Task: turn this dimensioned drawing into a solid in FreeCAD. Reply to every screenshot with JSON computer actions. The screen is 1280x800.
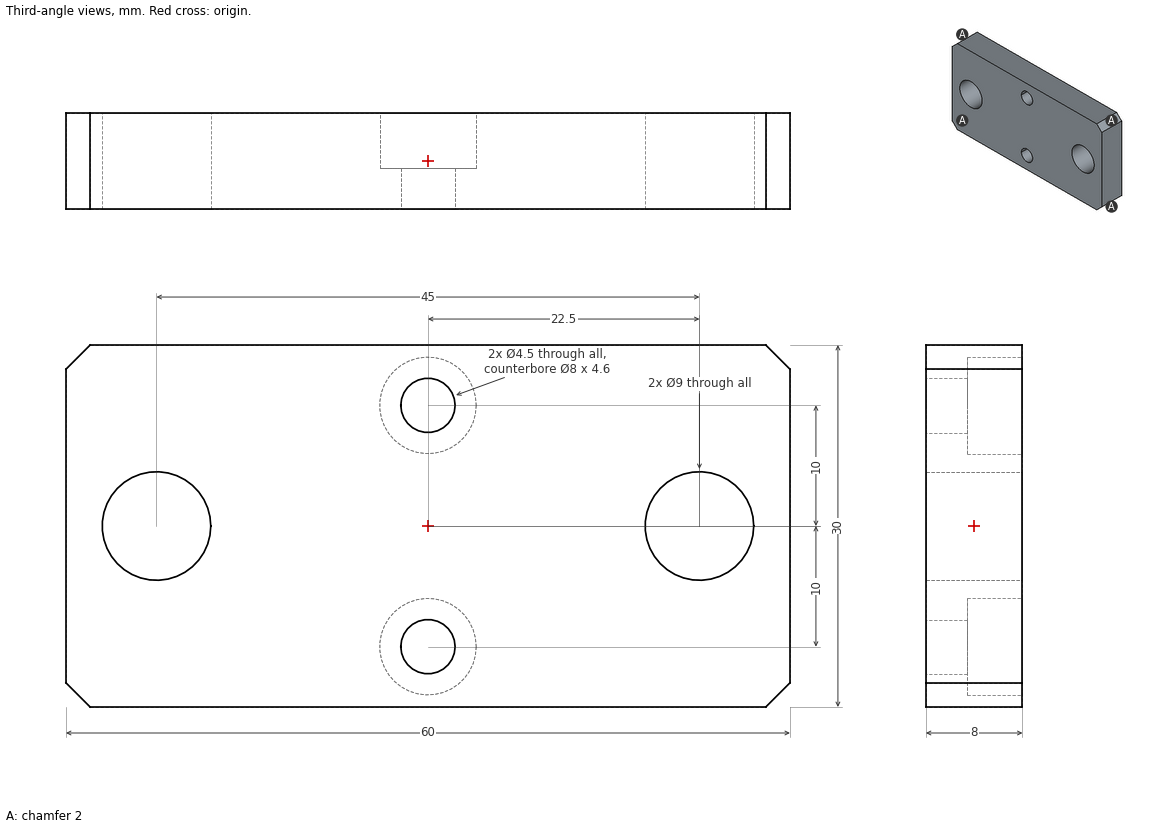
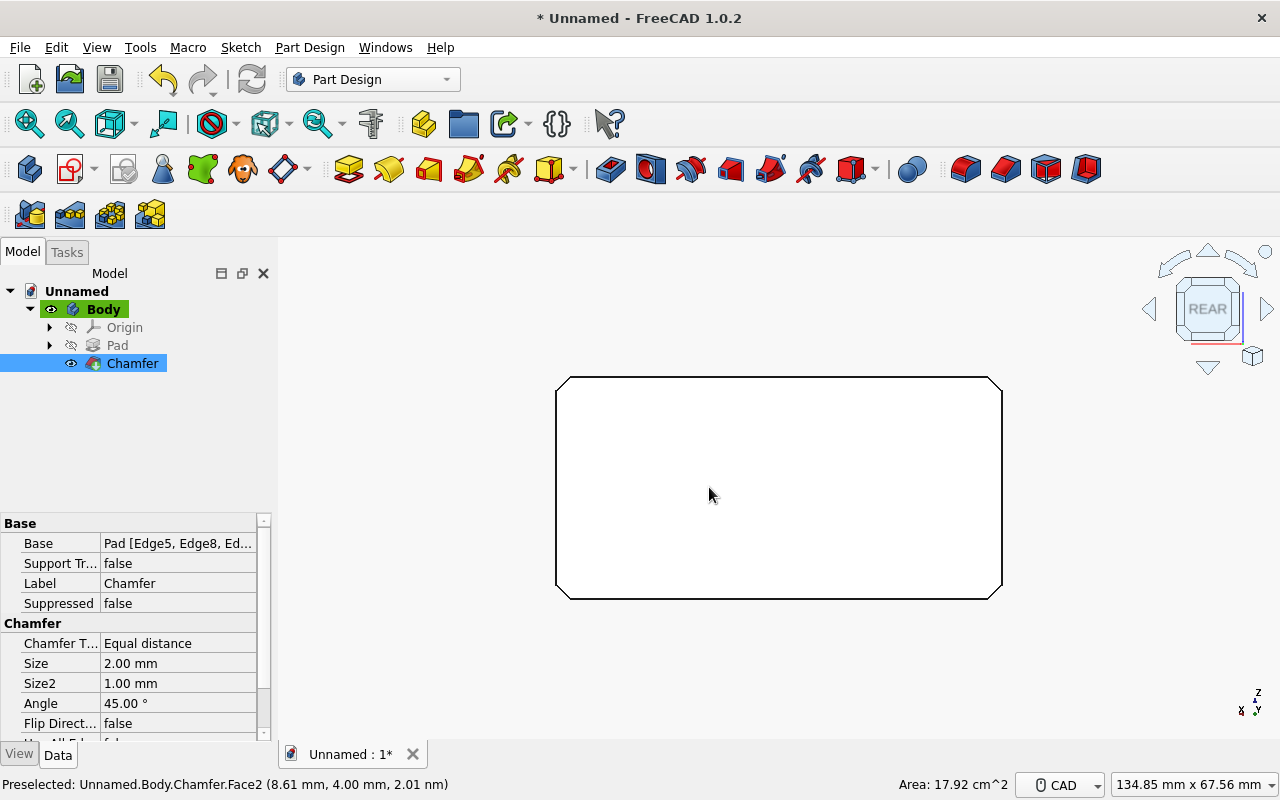
{"action": "left_click", "coordinate": [70, 170]}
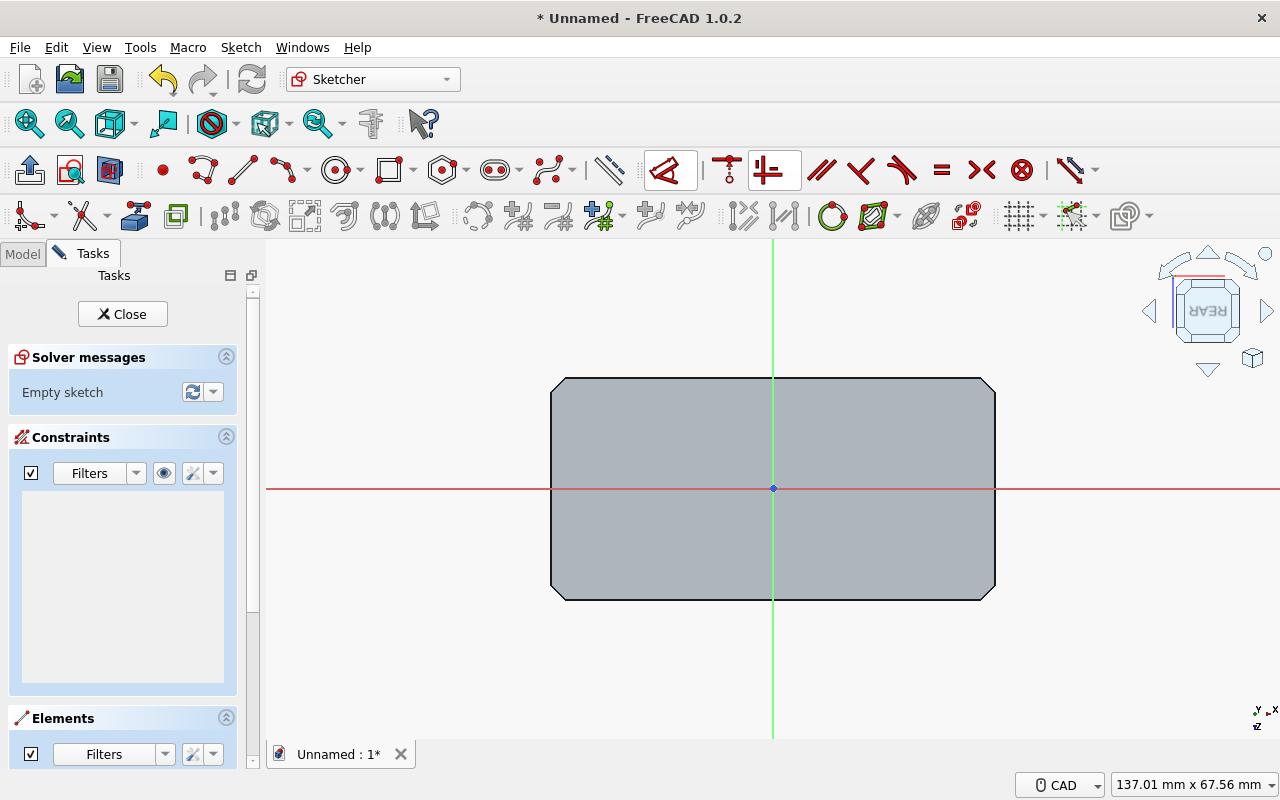
{"action": "scroll", "coordinate": [856, 489], "scroll_direction": "up", "scroll_amount": 3}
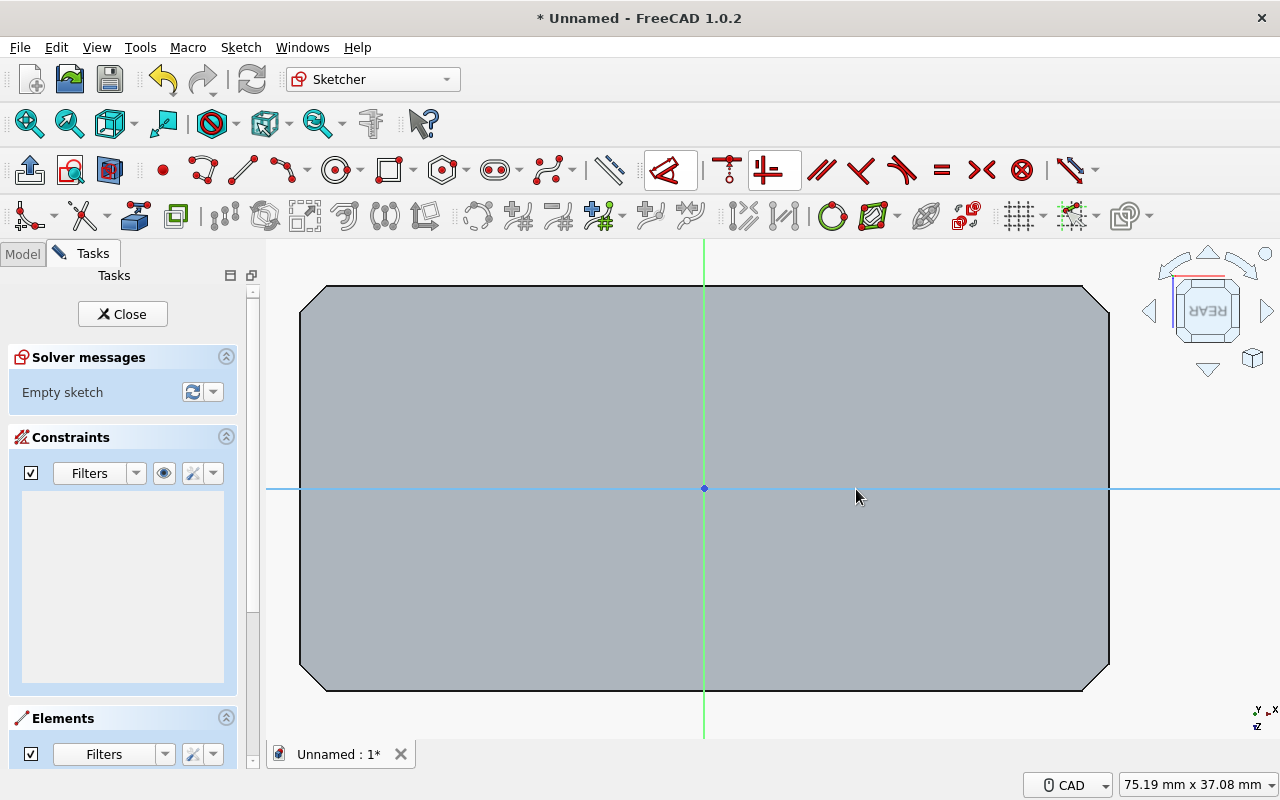
{"action": "left_click", "coordinate": [336, 170]}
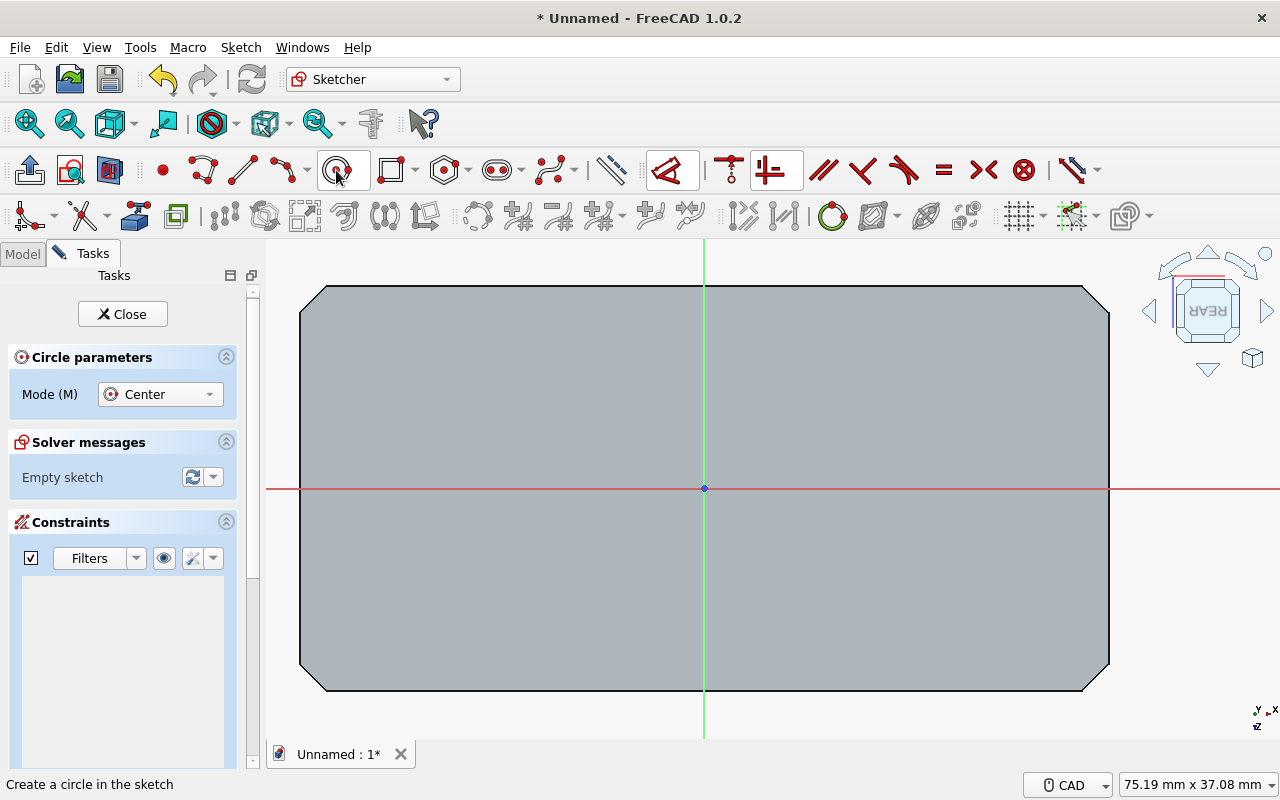
{"action": "left_click", "coordinate": [704, 623]}
{"action": "left_click", "coordinate": [726, 602]}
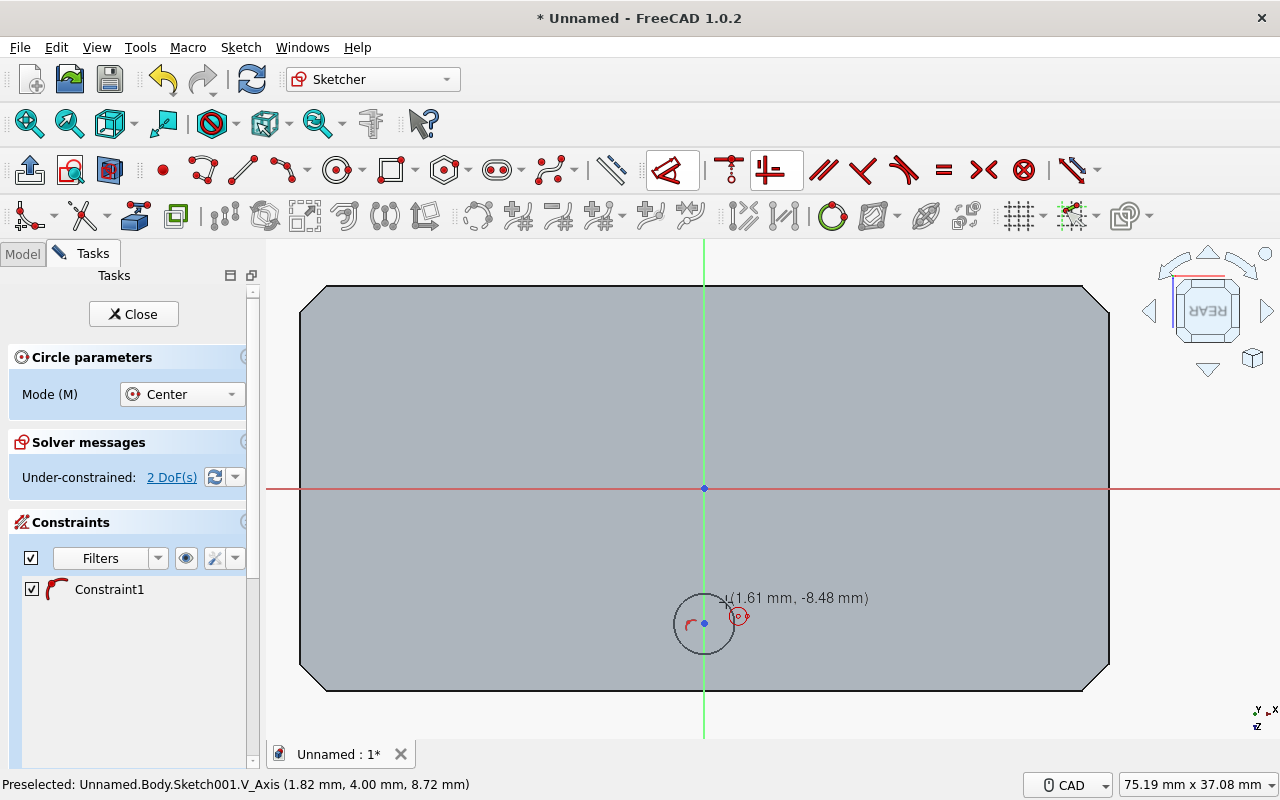
{"action": "left_click", "coordinate": [704, 354]}
{"action": "left_click", "coordinate": [726, 332]}
{"action": "key", "text": "Escape"}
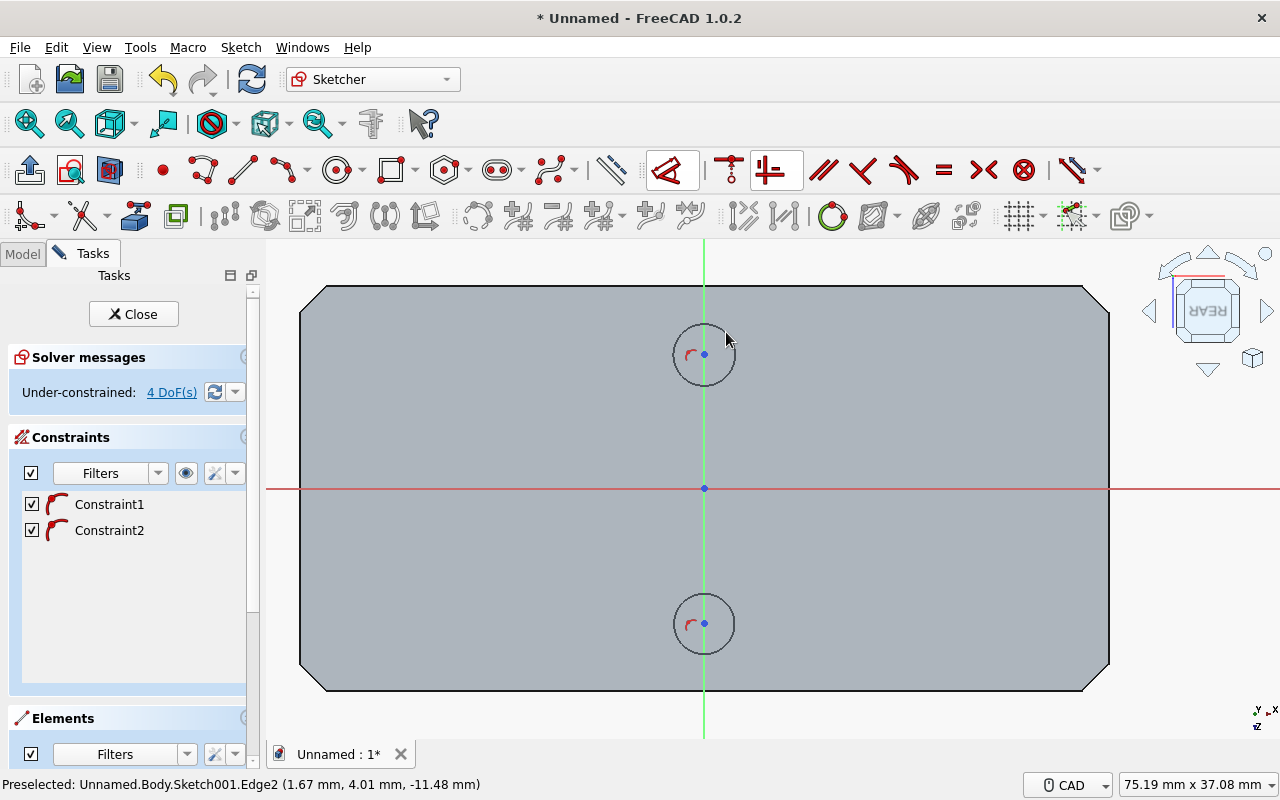
{"action": "left_click", "coordinate": [726, 603]}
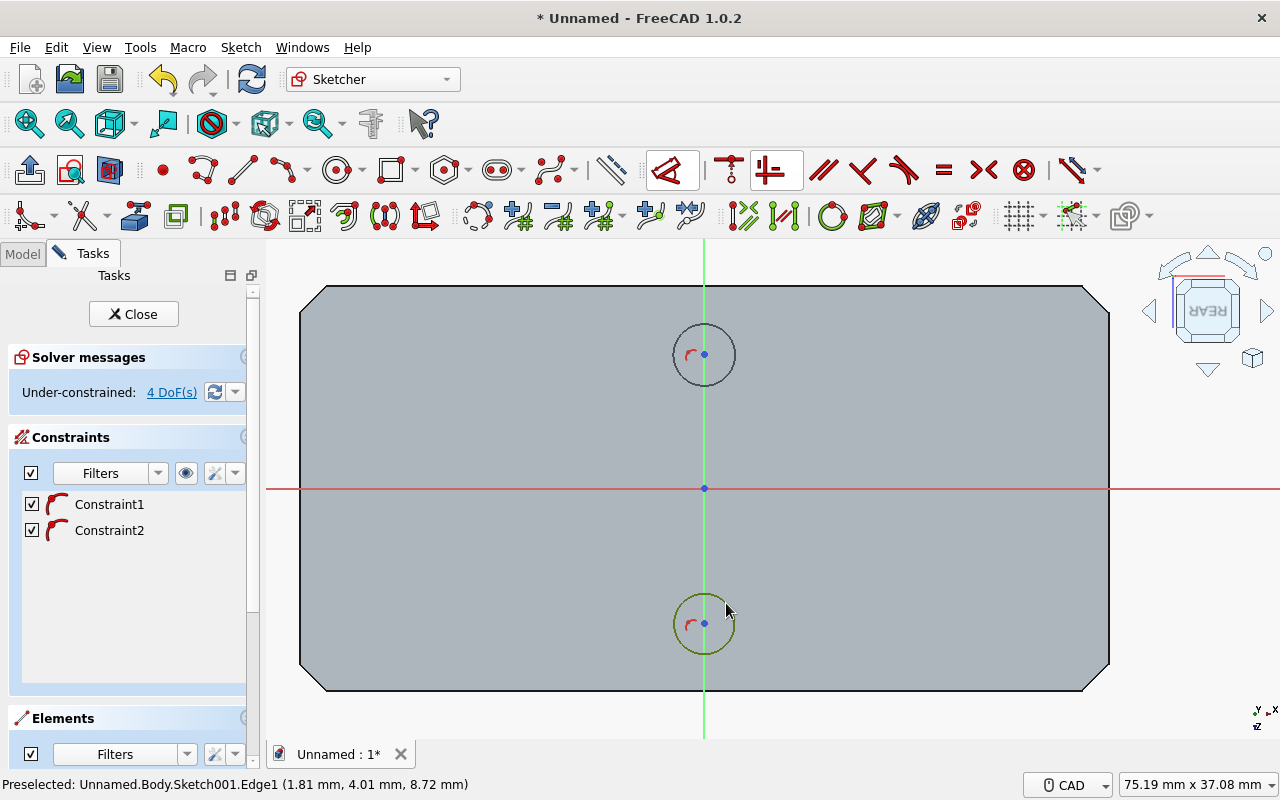
{"action": "left_click", "coordinate": [726, 333]}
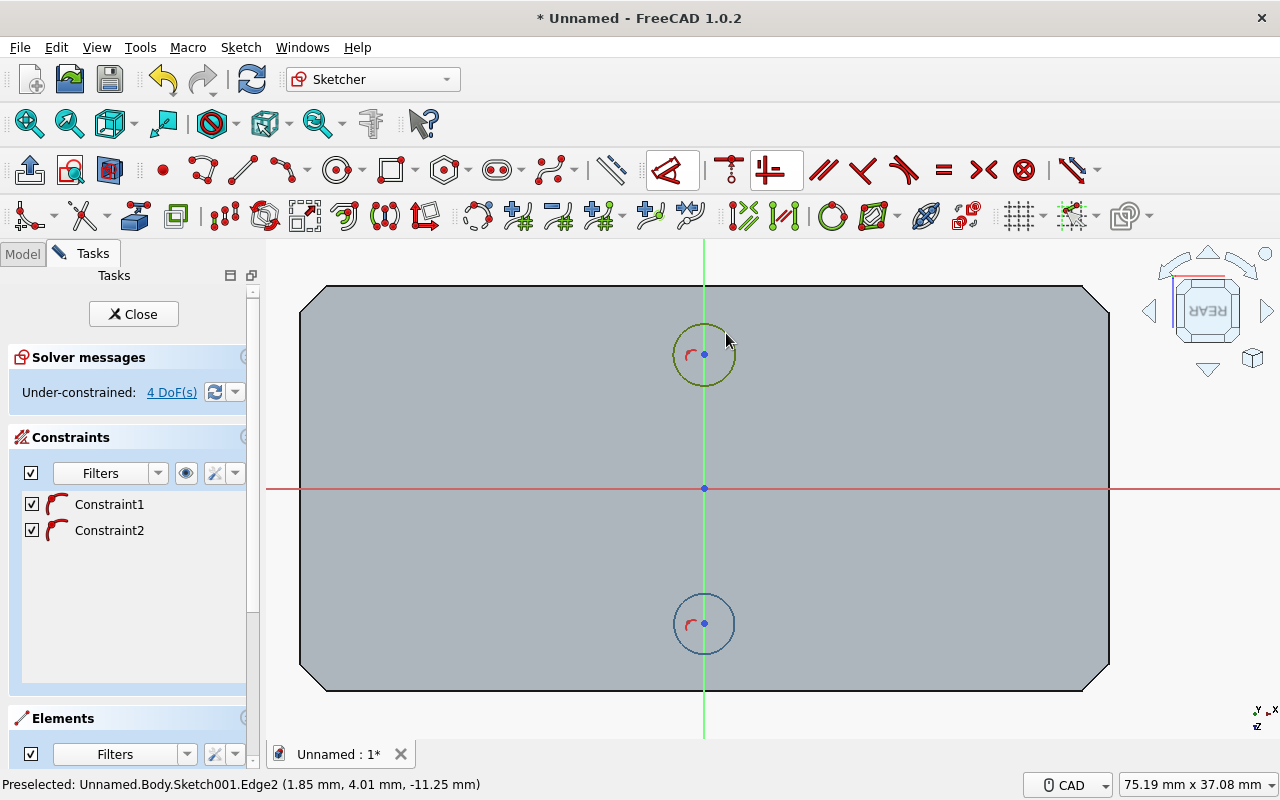
{"action": "left_click", "coordinate": [944, 170]}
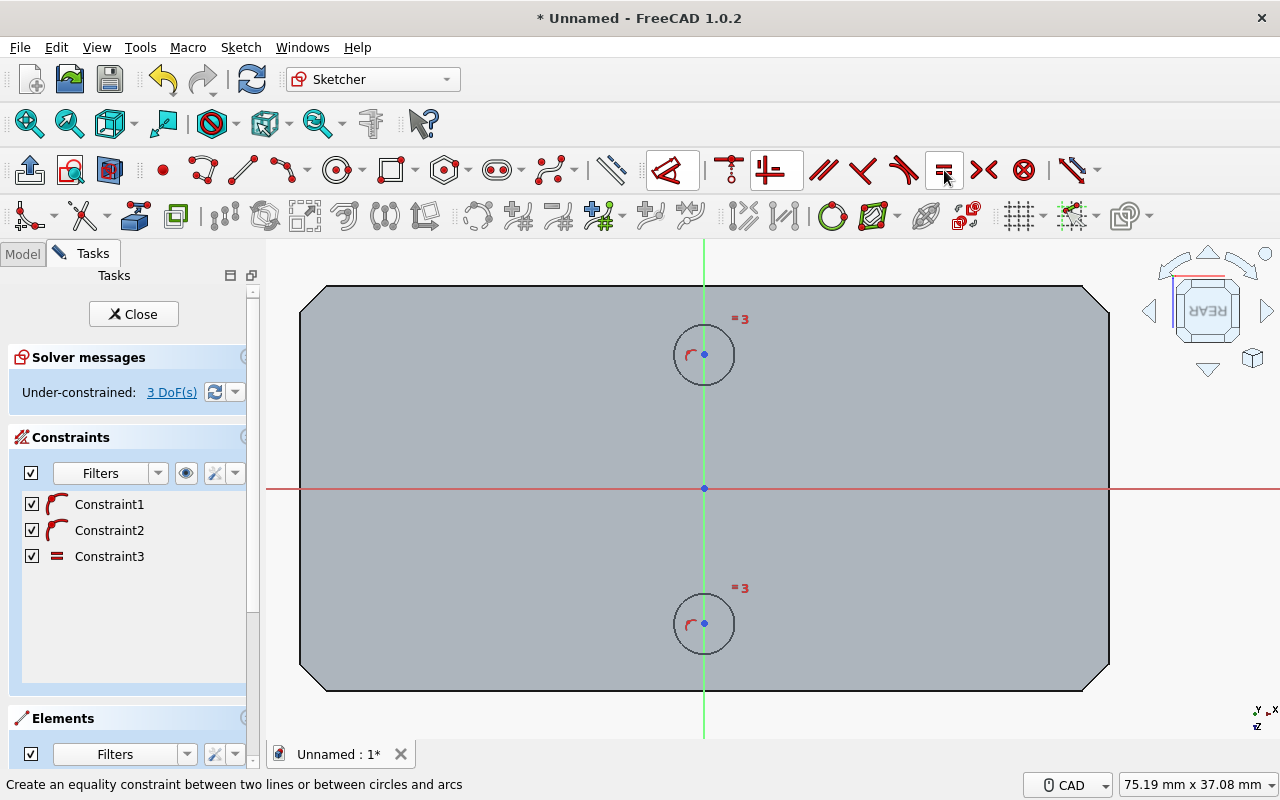
{"action": "left_click", "coordinate": [726, 603]}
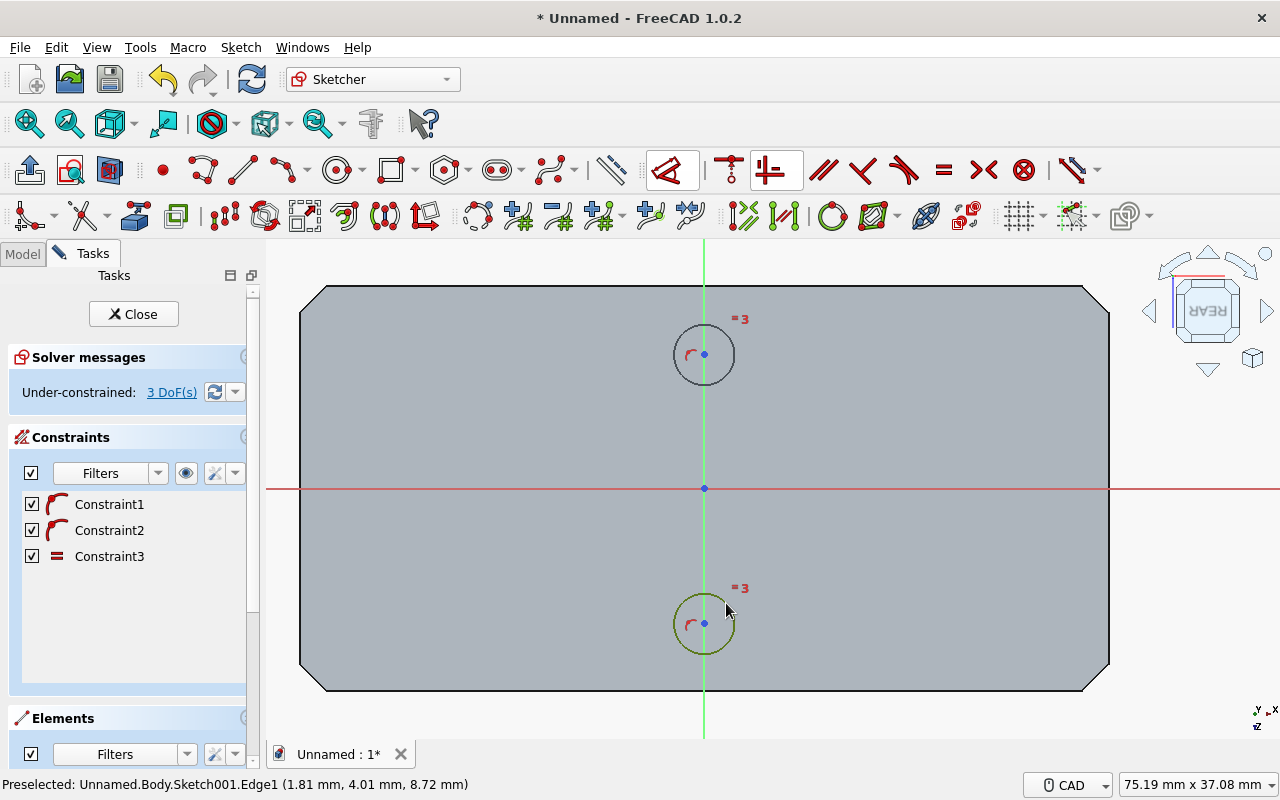
{"action": "key", "text": "k o"}